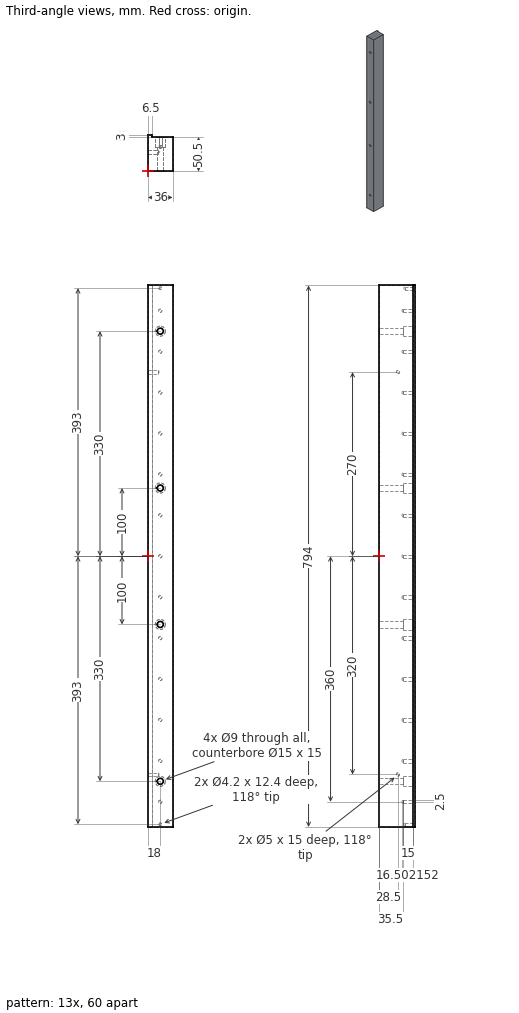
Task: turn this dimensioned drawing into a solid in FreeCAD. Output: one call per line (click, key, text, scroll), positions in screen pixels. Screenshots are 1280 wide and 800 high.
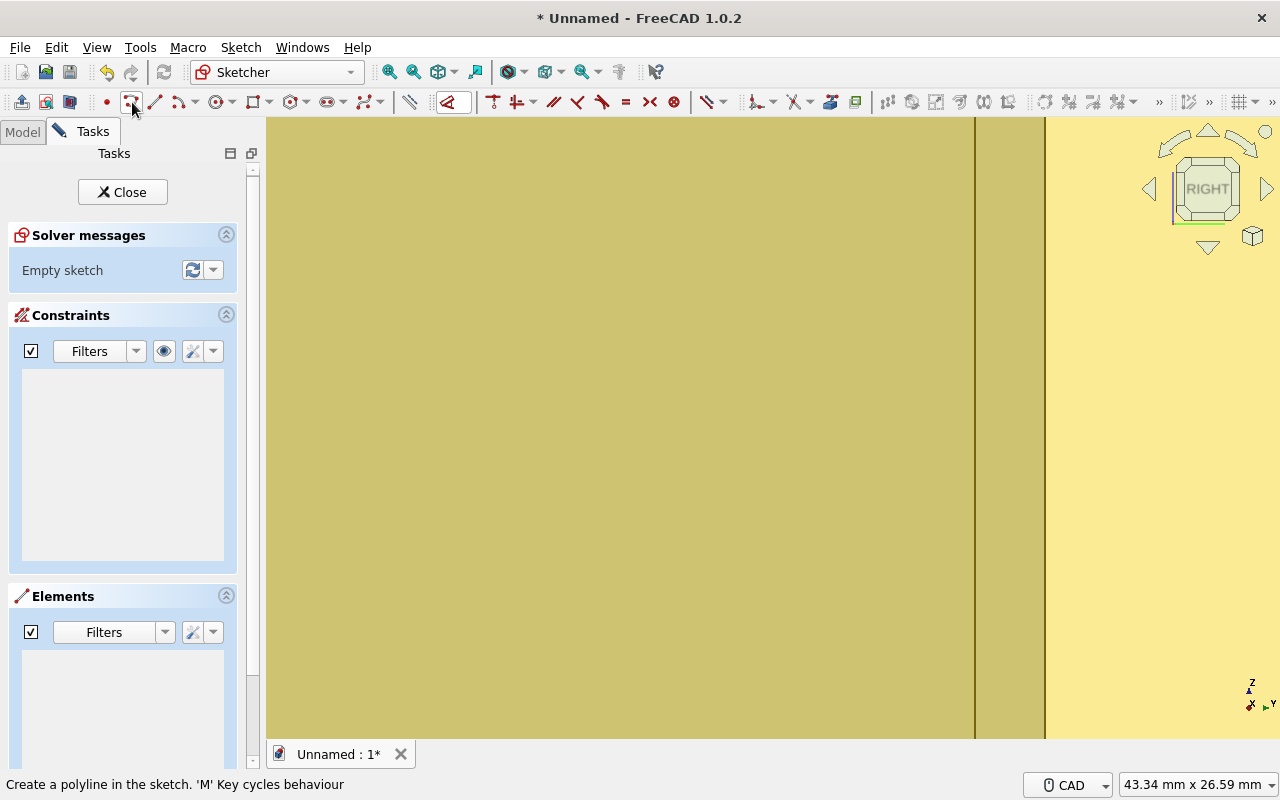
click(624, 568)
click(589, 626)
click(975, 626)
click(975, 568)
click(624, 569)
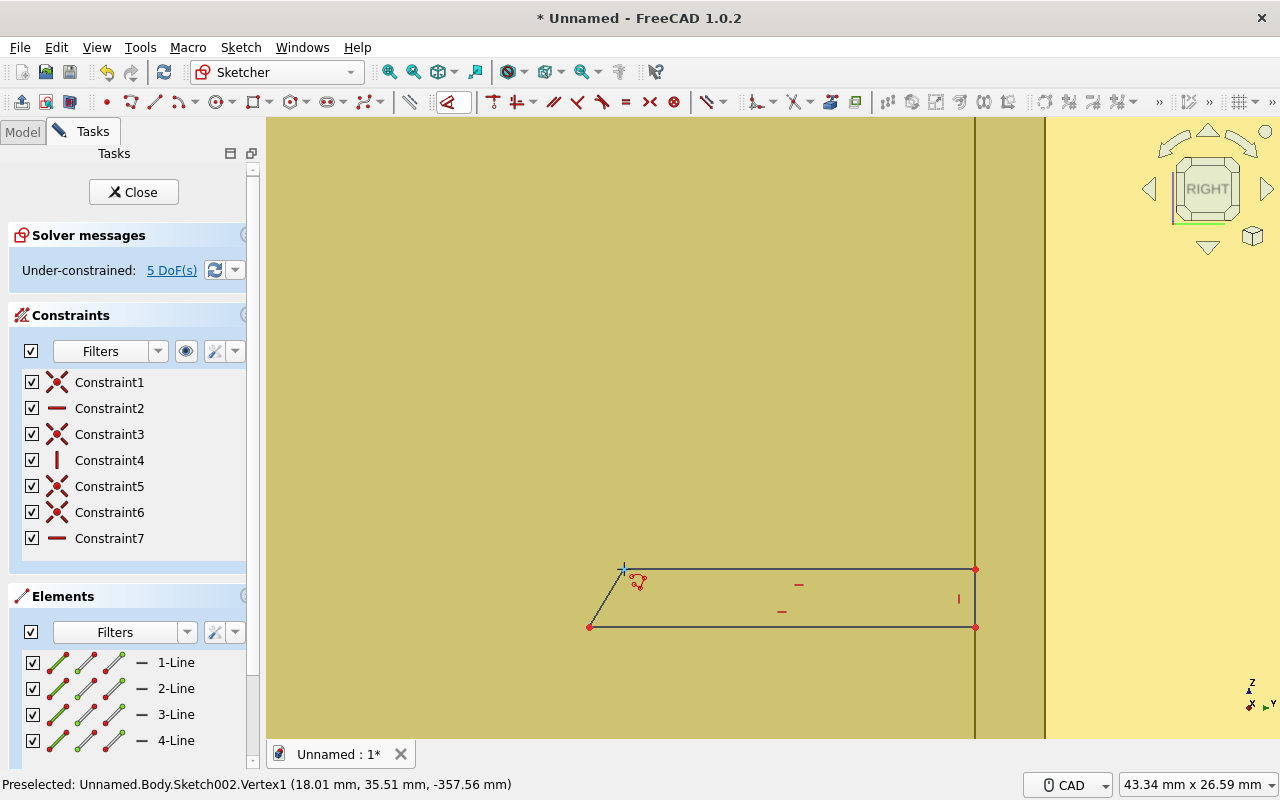
click(156, 102)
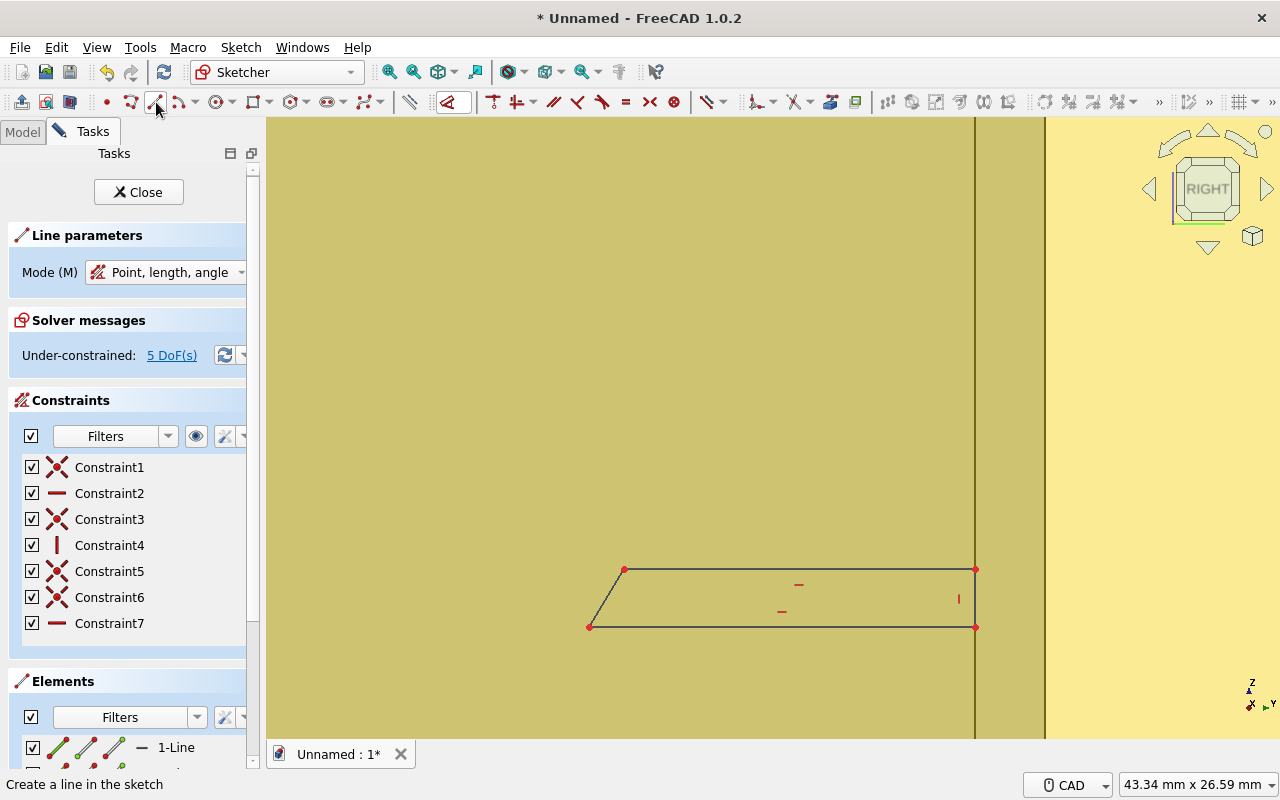
click(550, 626)
click(434, 626)
key(Escape)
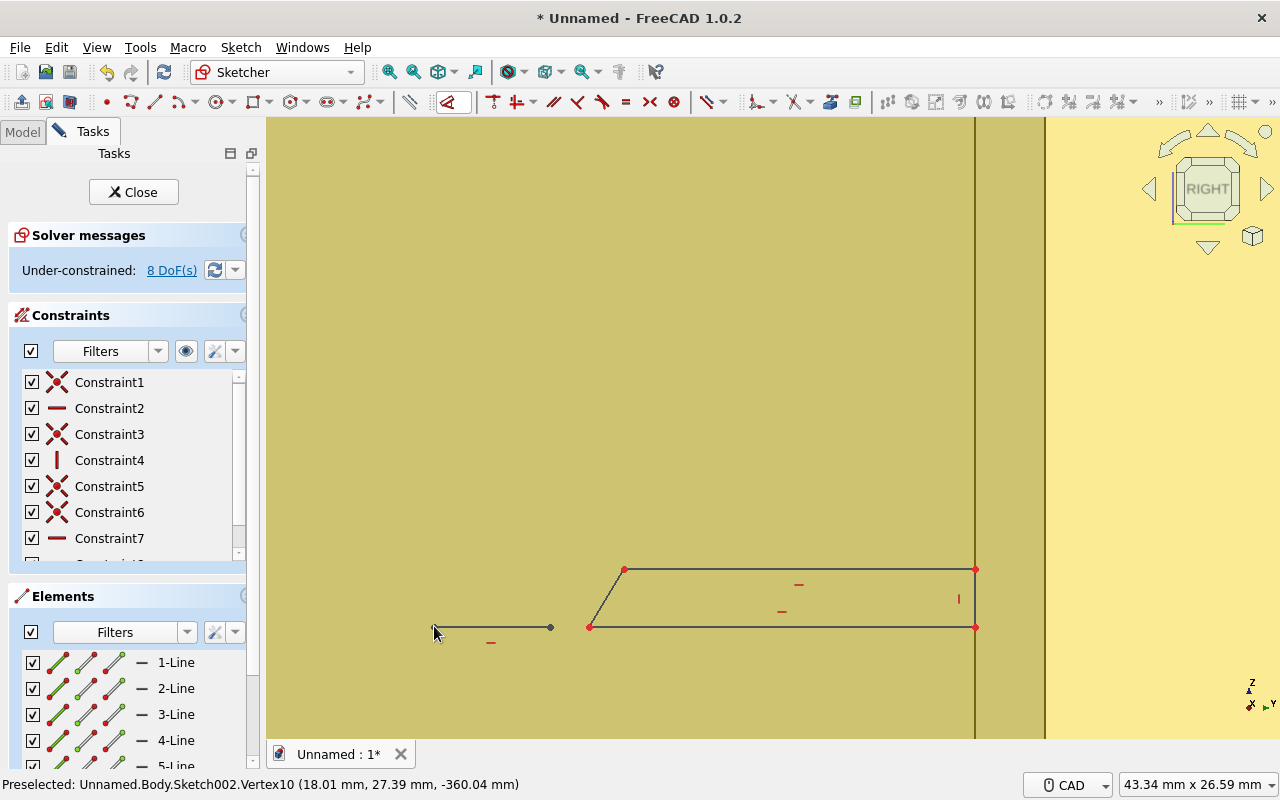
click(515, 627)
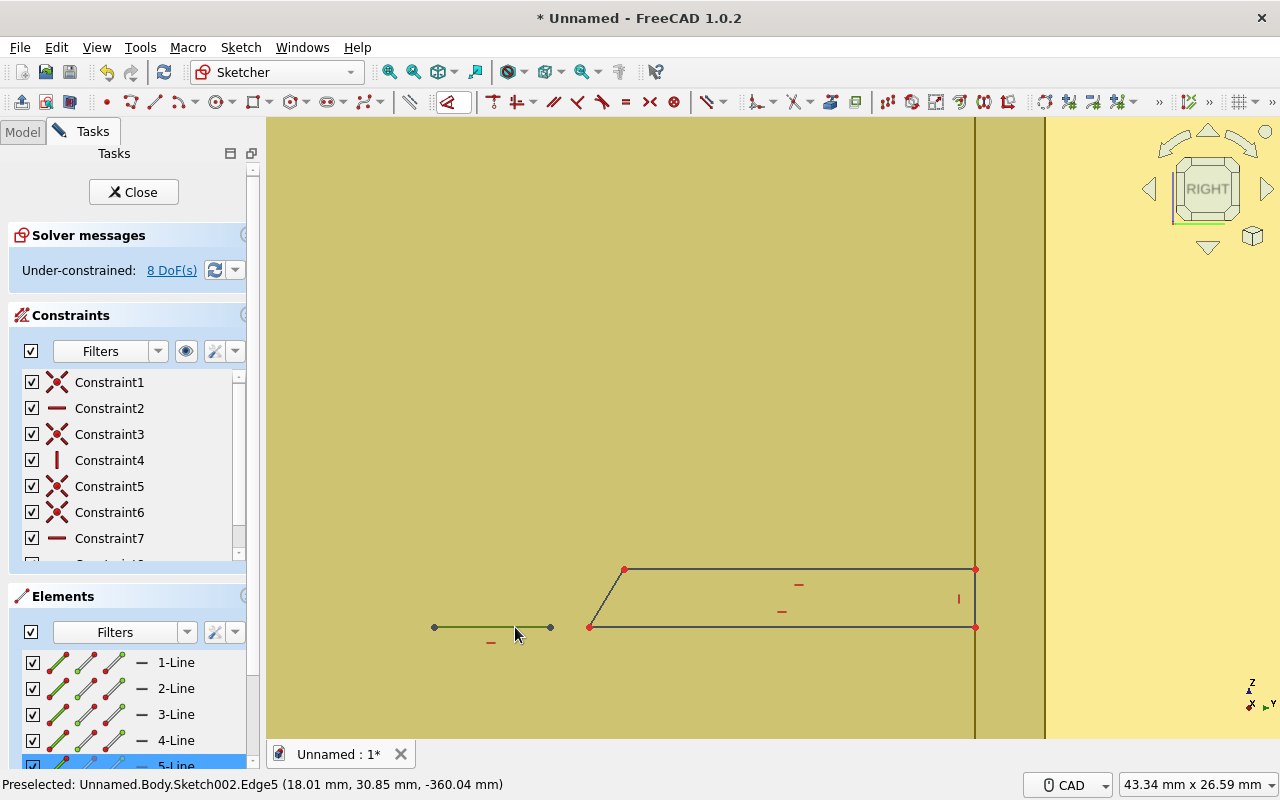
click(410, 102)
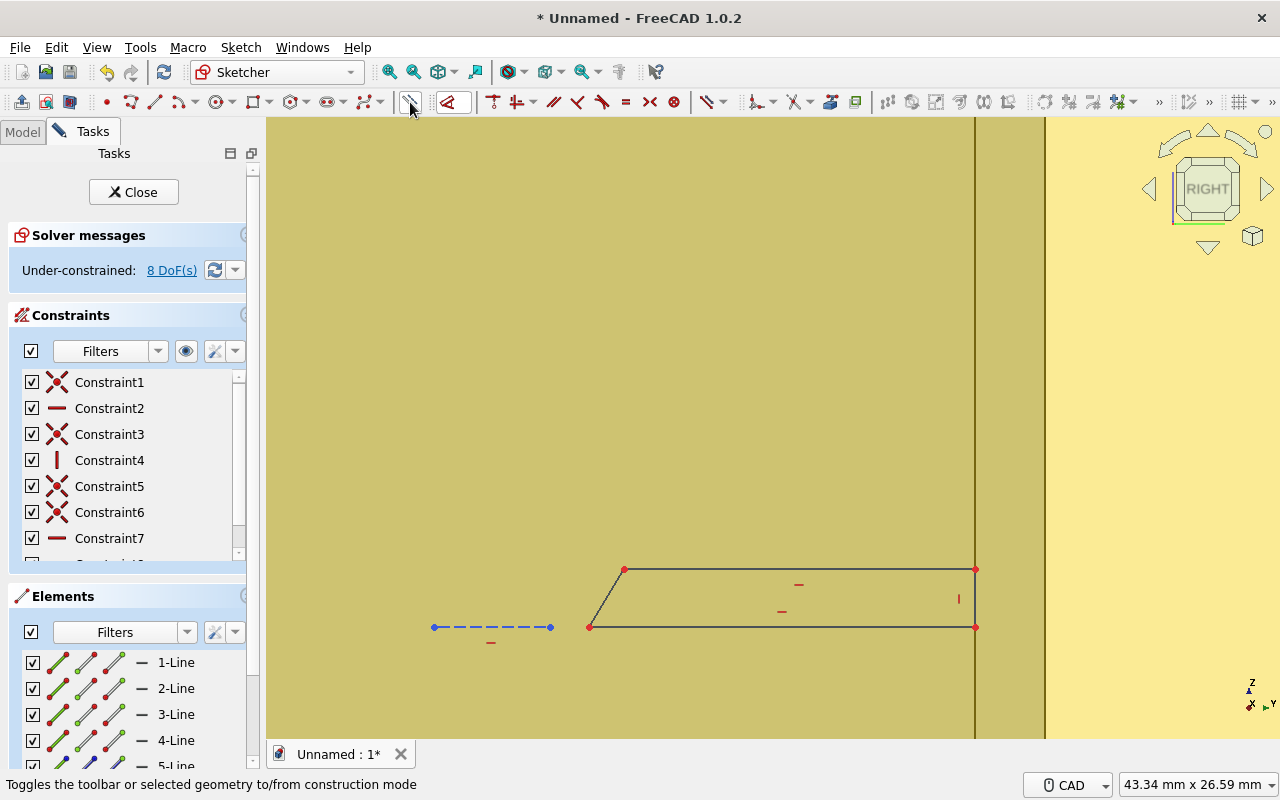
click(870, 569)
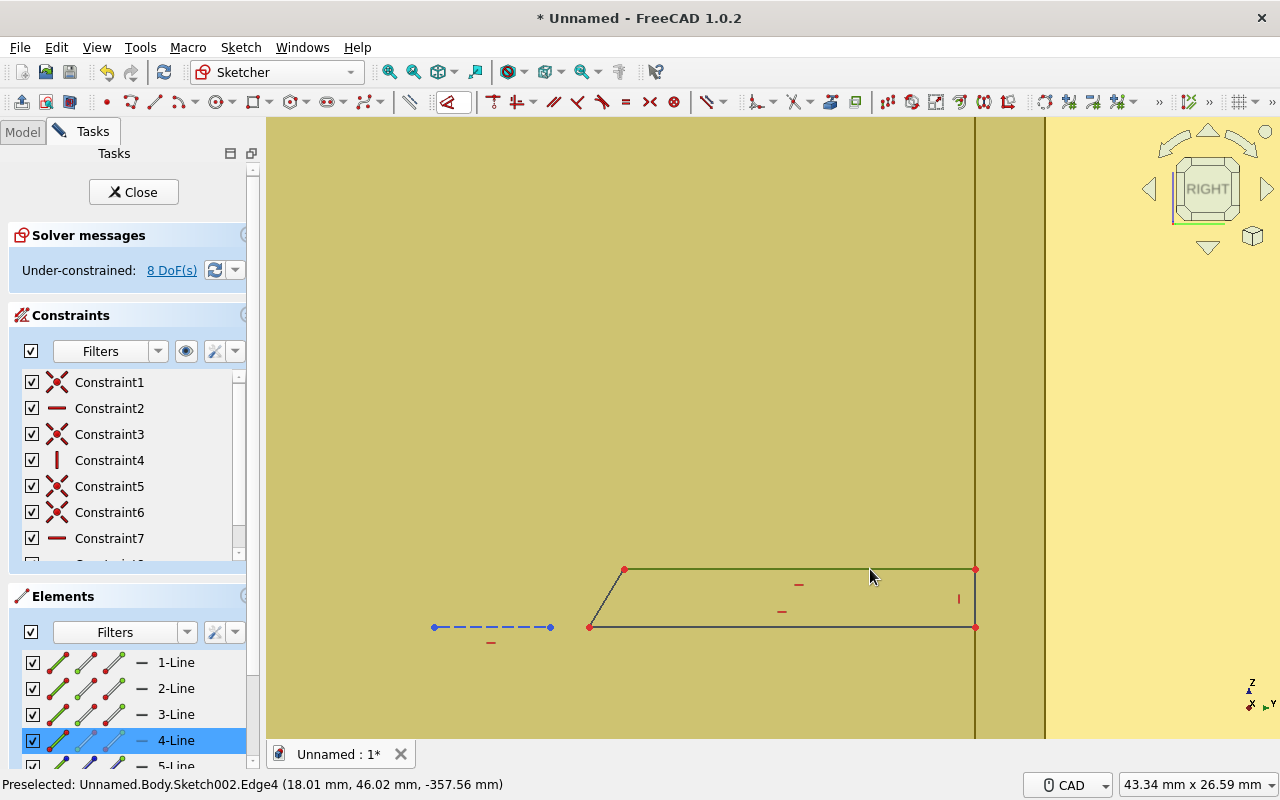
key(l)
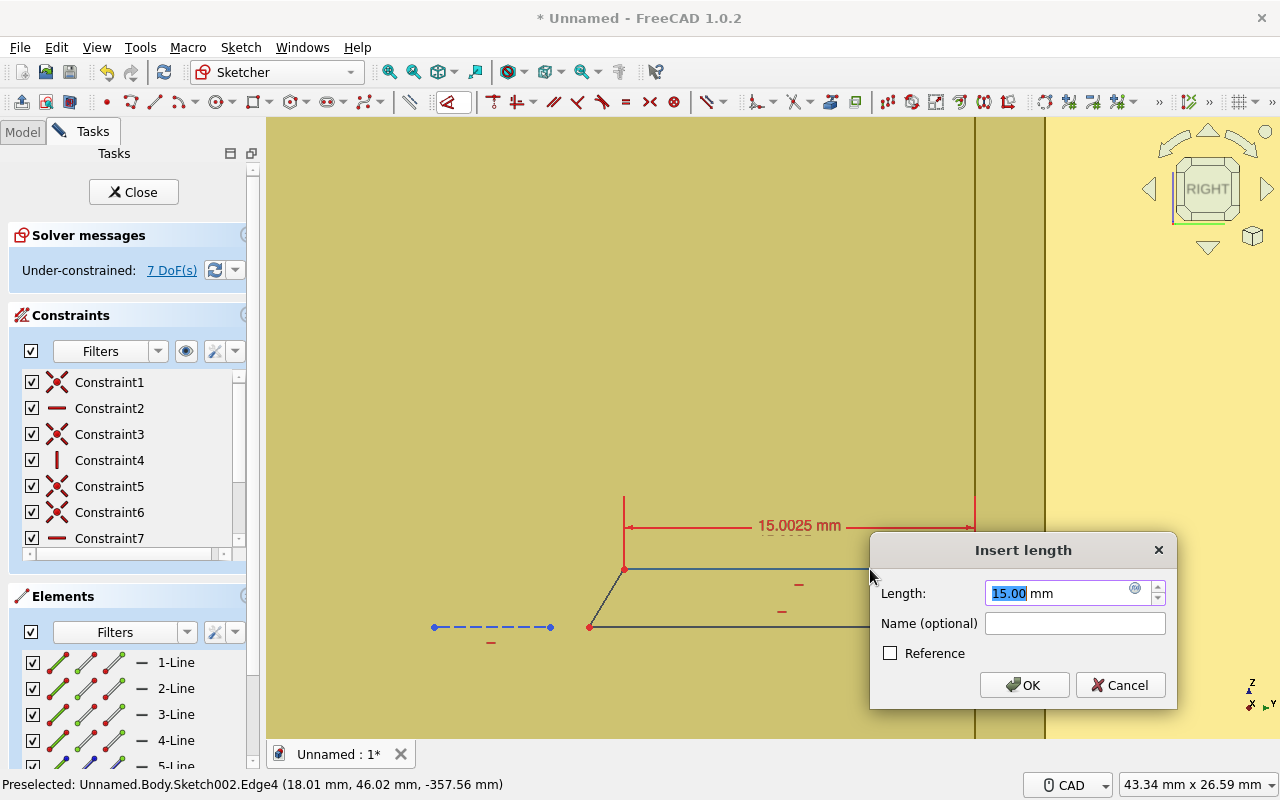
text(15)
key(Return)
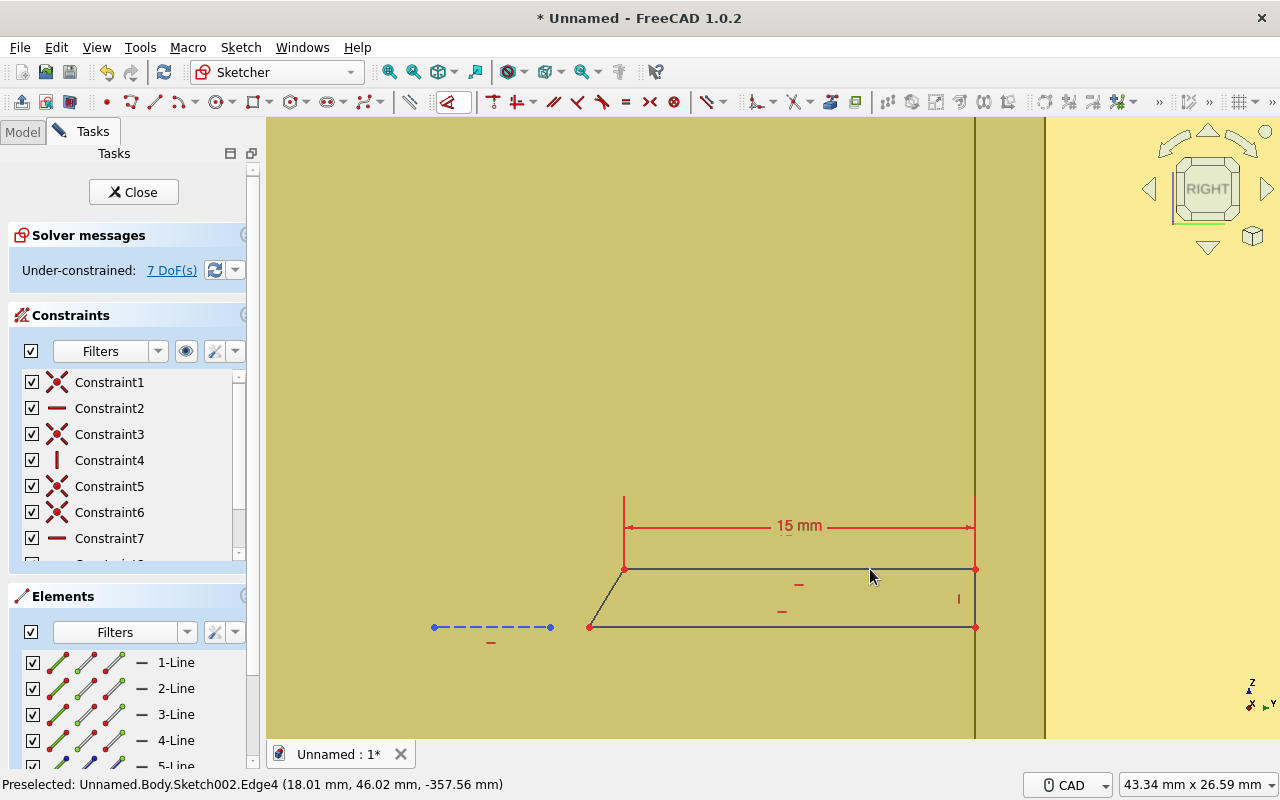
click(975, 610)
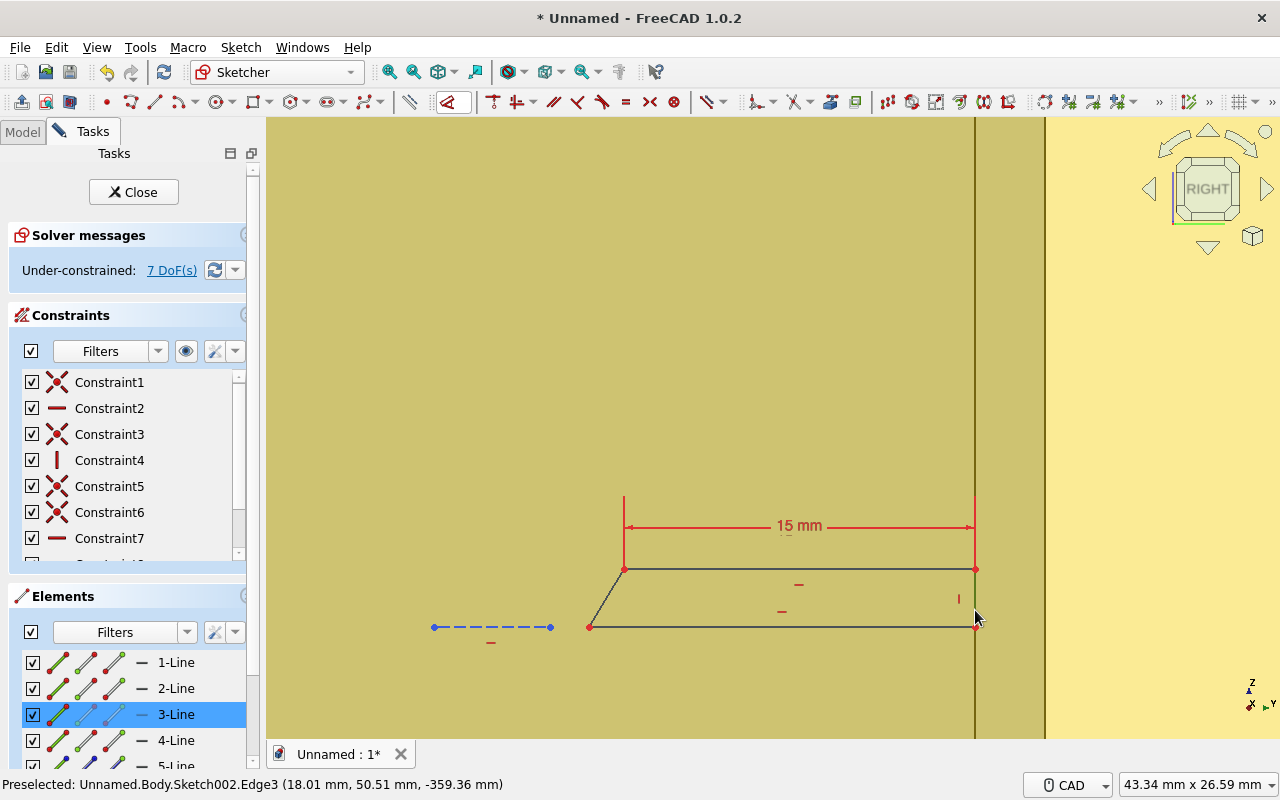
click(466, 102)